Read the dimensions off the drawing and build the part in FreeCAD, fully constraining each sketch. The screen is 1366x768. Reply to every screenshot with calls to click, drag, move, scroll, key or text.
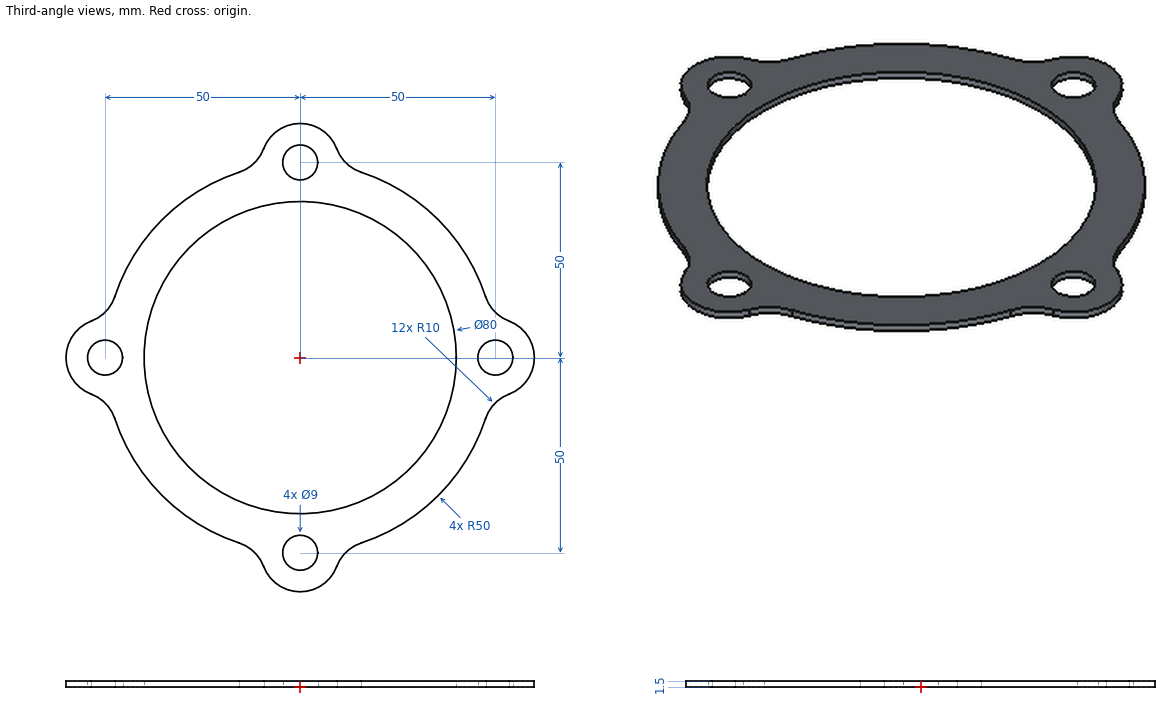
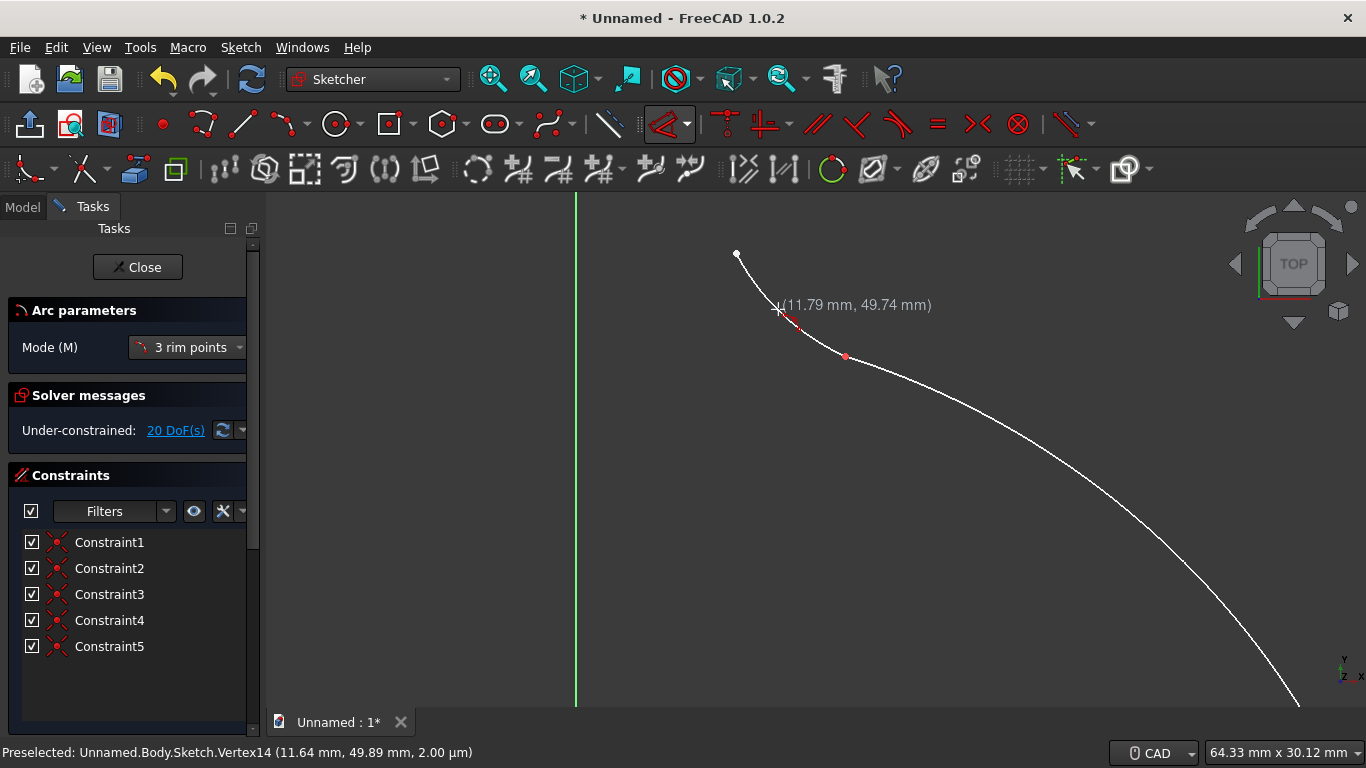
scroll(781, 309, down, 9)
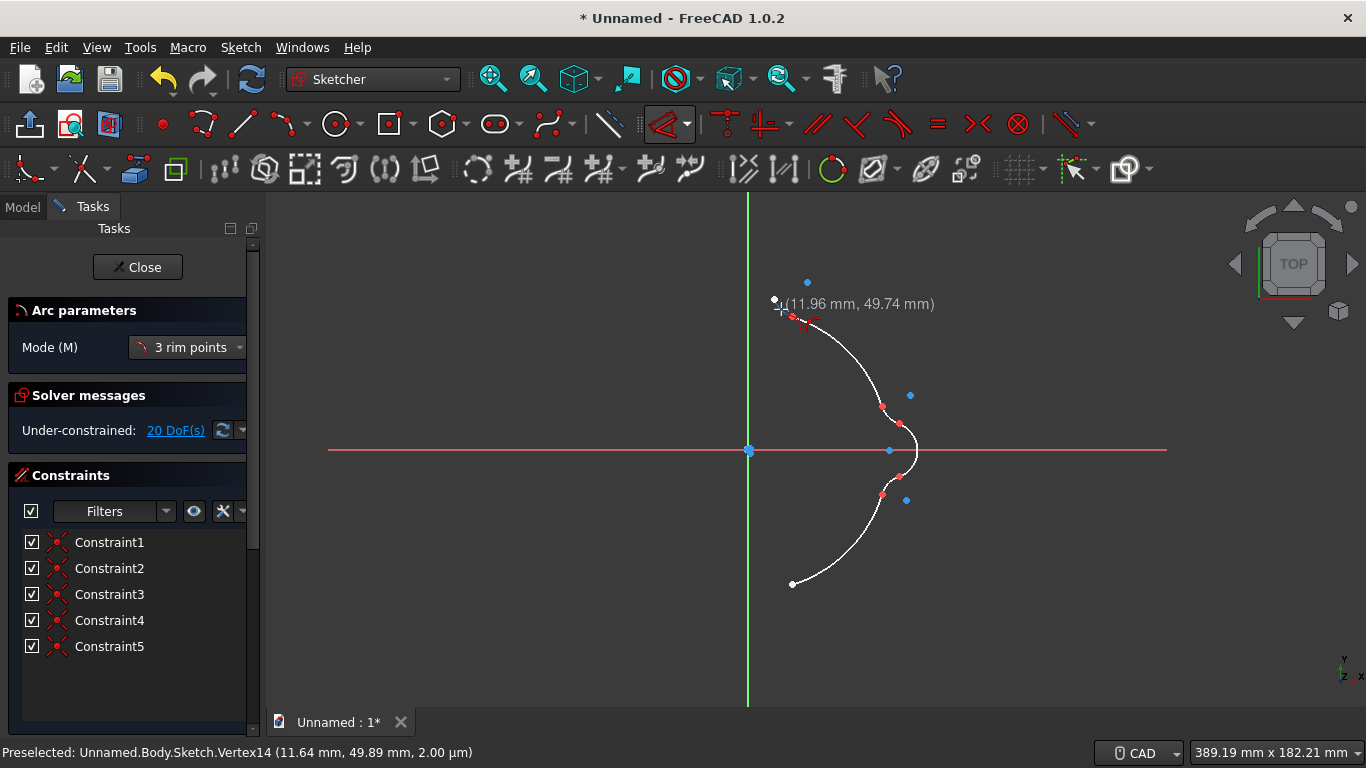
click(774, 300)
click(721, 299)
click(734, 284)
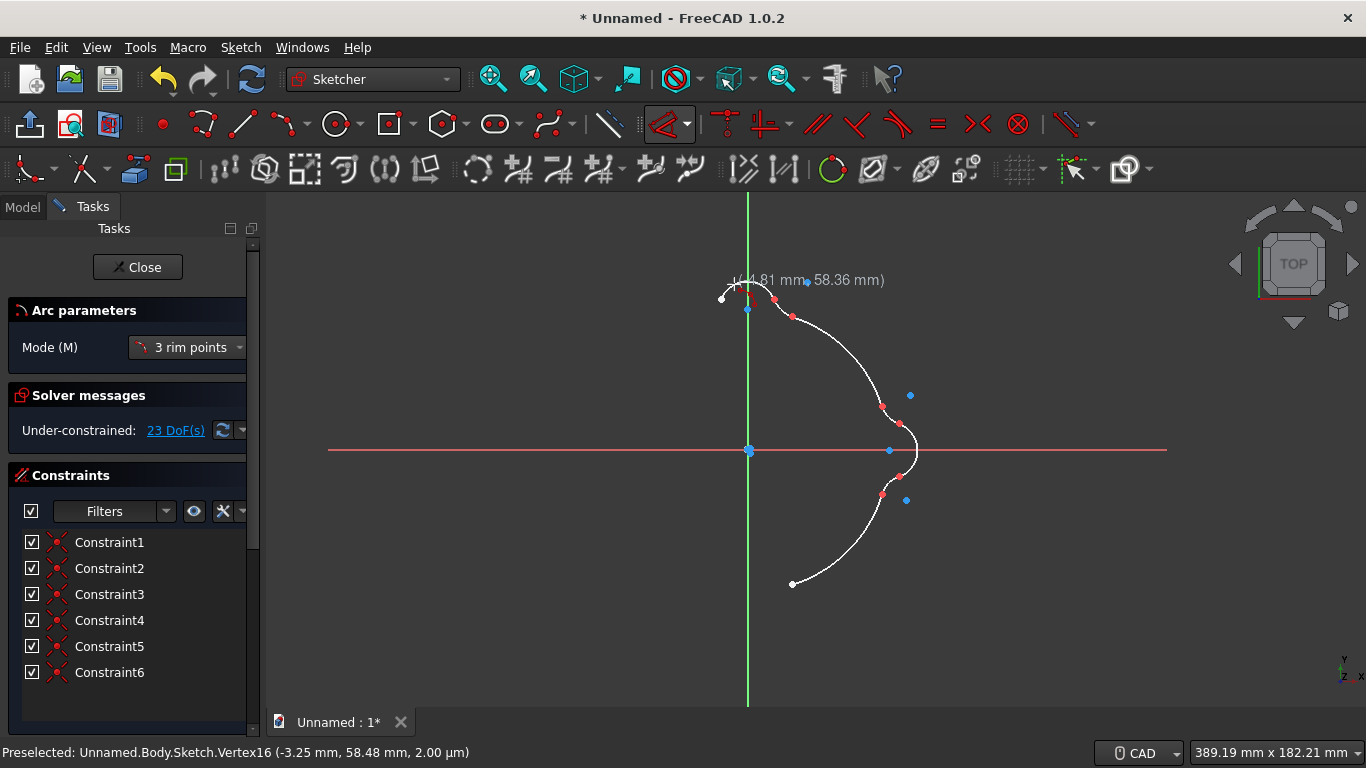
click(721, 300)
click(703, 316)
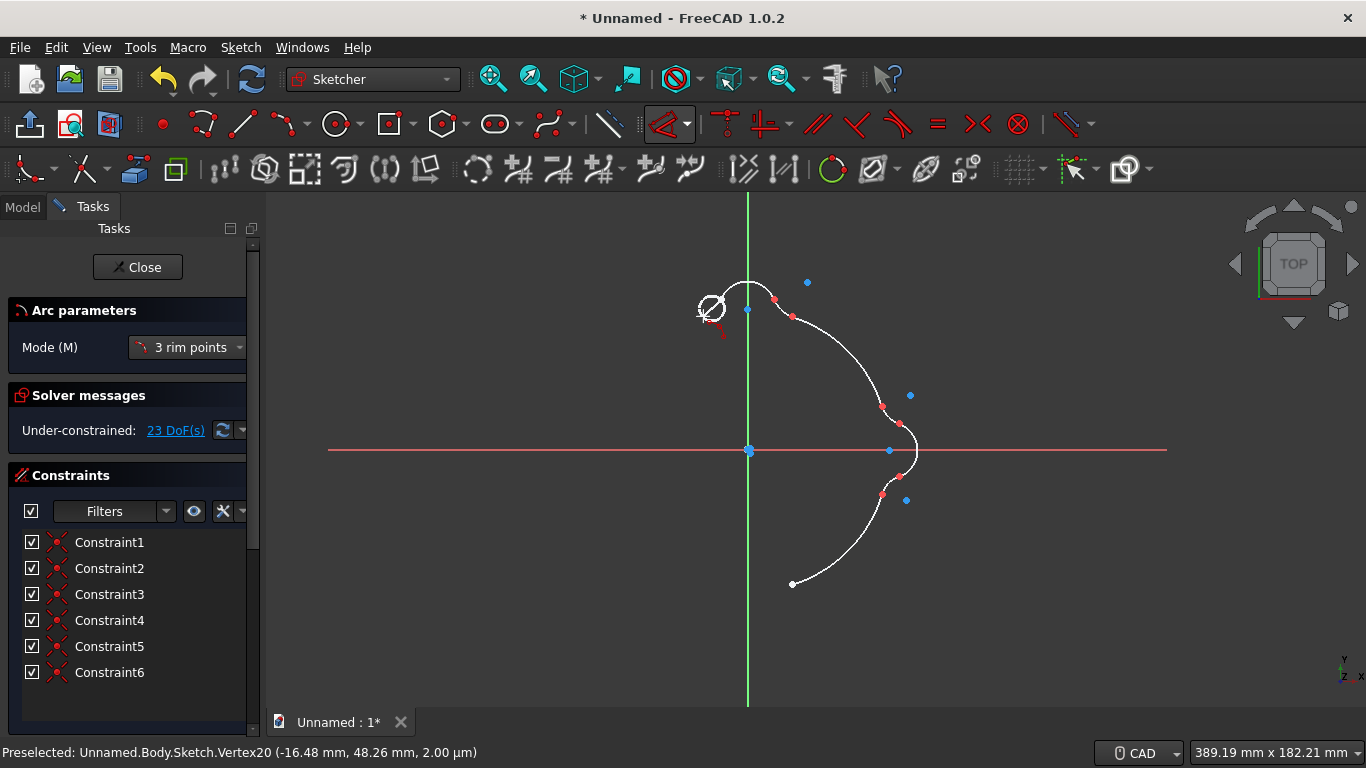
scroll(714, 309, up, 9)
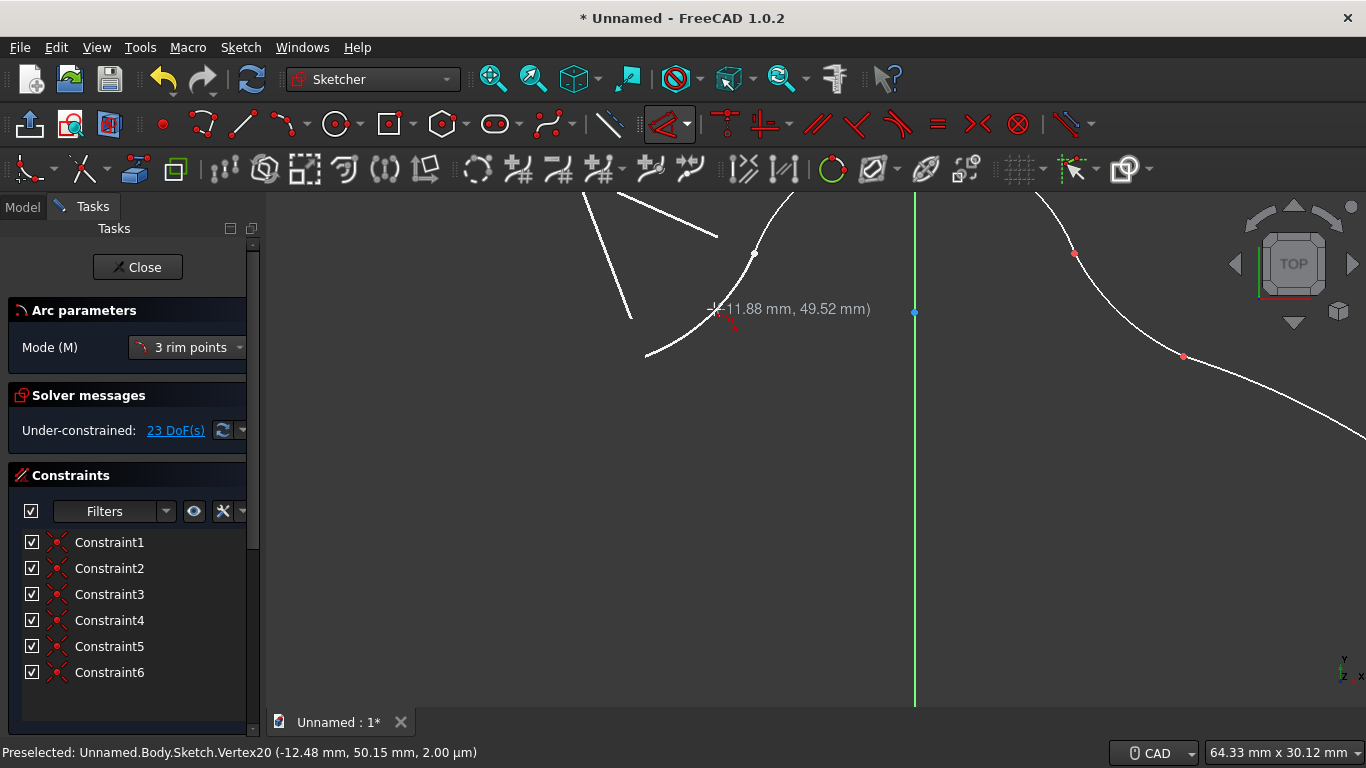
click(713, 309)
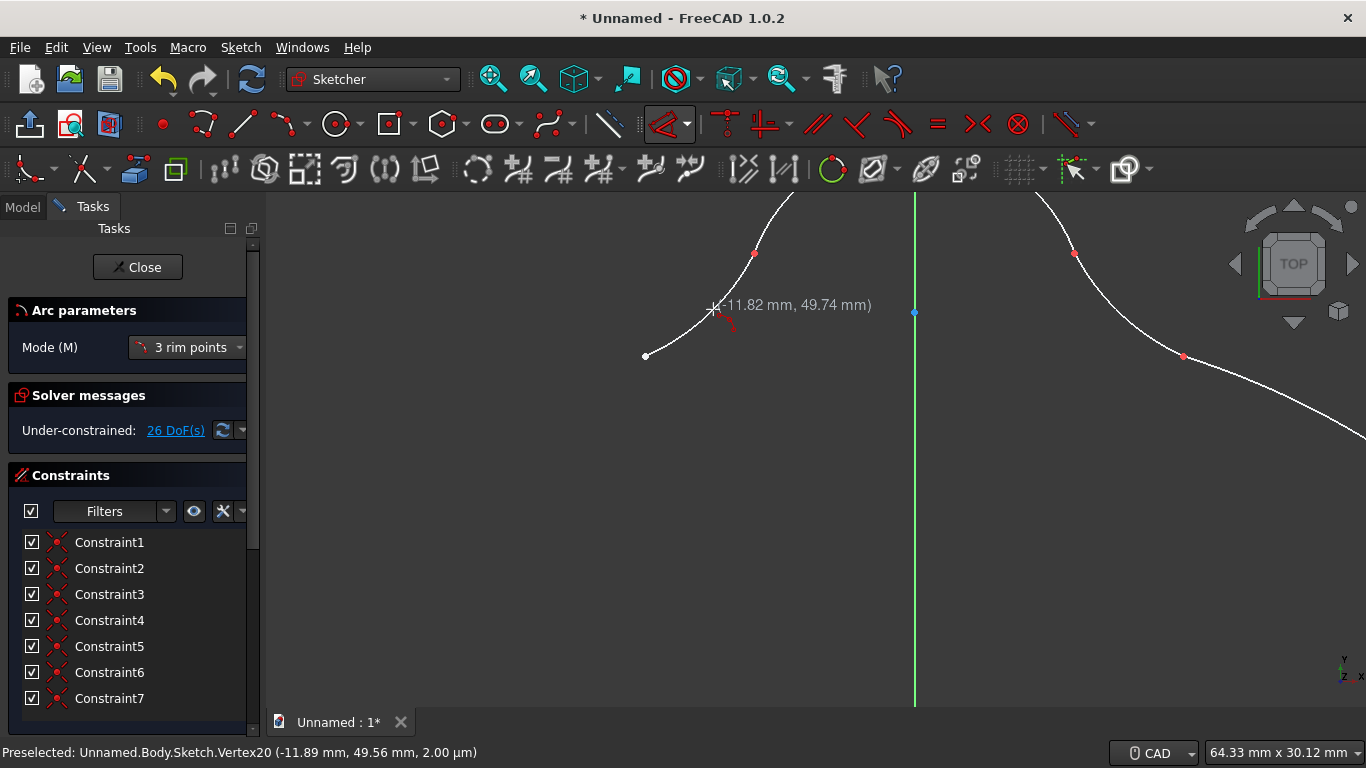
scroll(714, 309, down, 9)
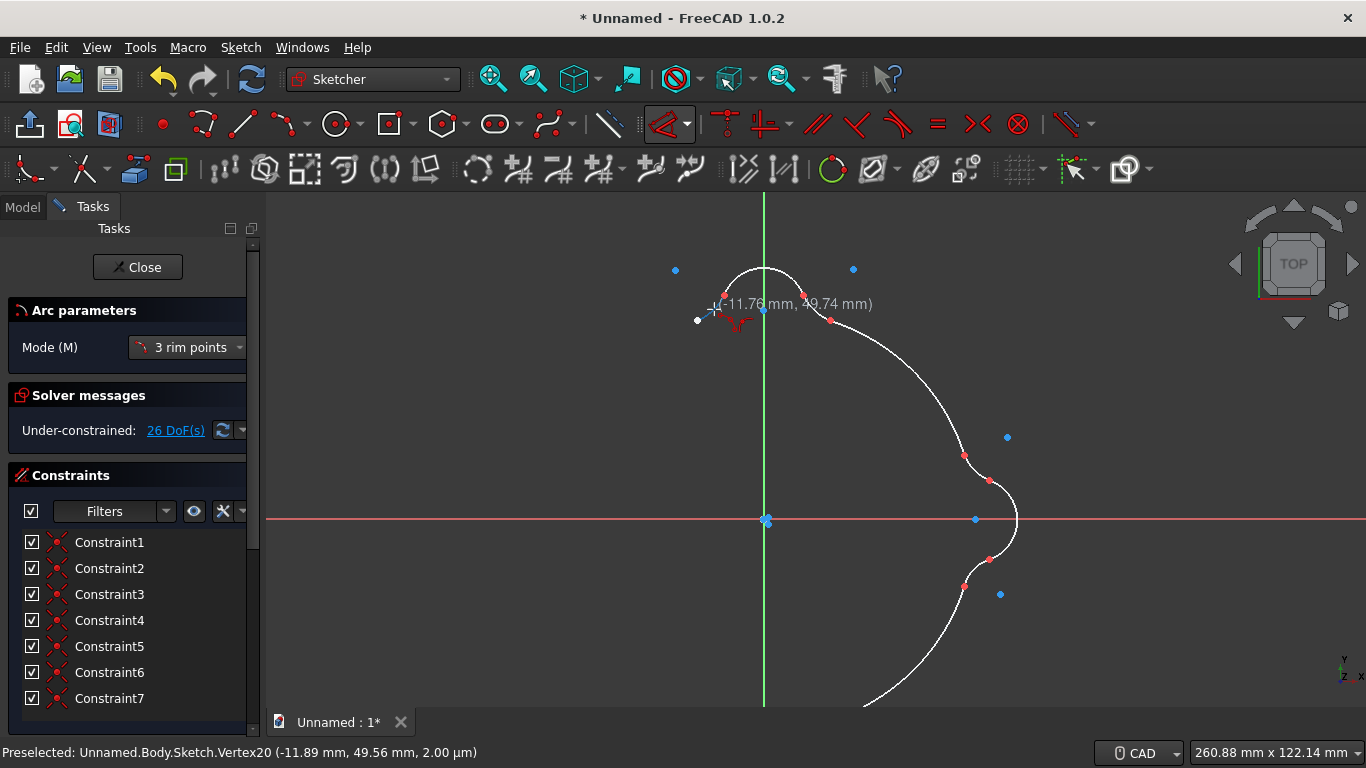
click(703, 317)
click(613, 406)
click(648, 350)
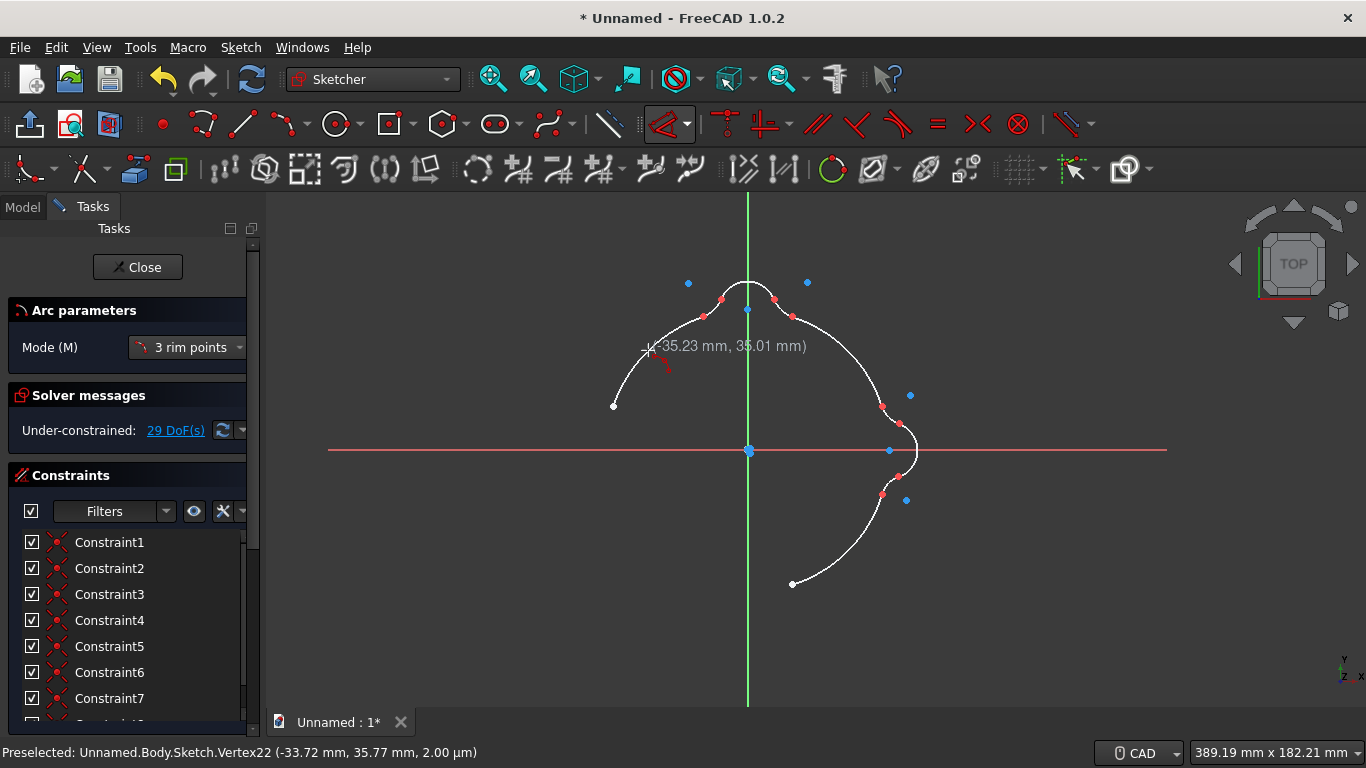
click(613, 407)
click(596, 423)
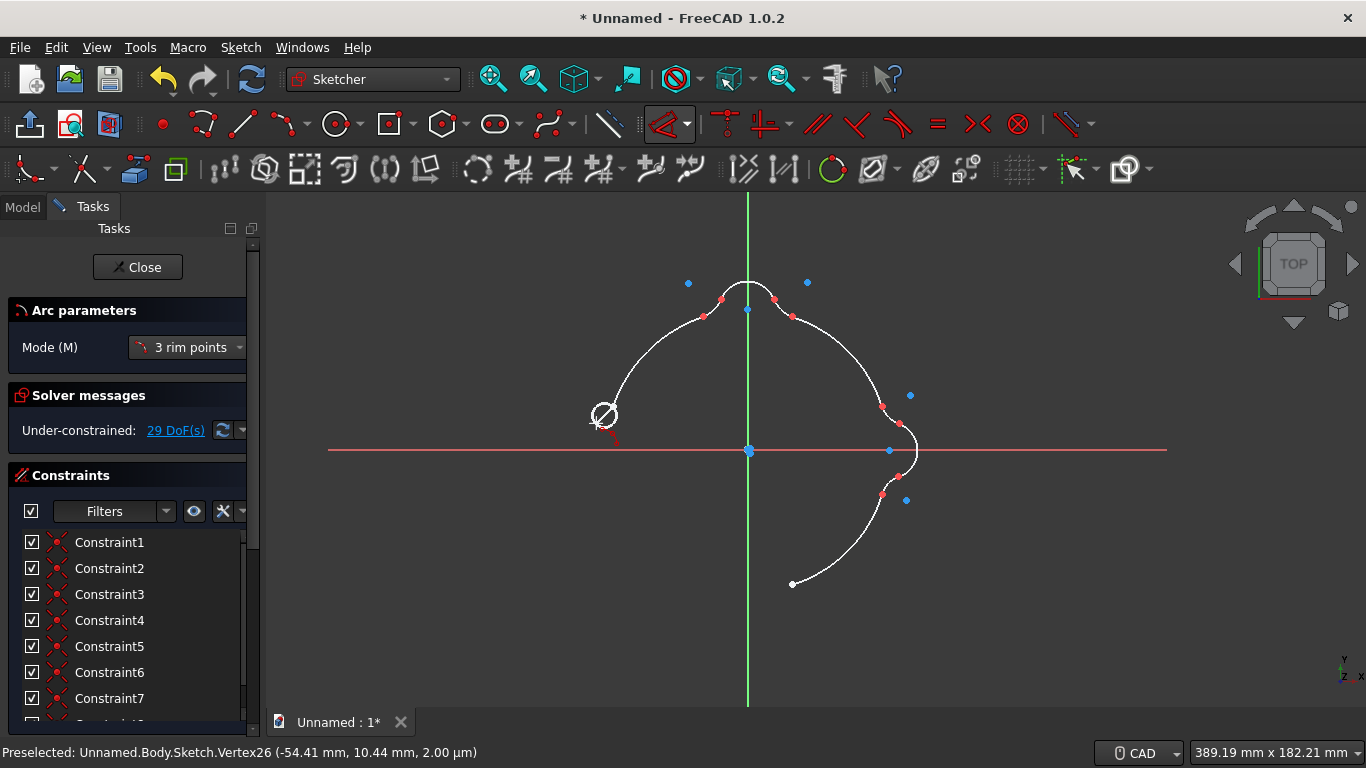
scroll(607, 417, up, 9)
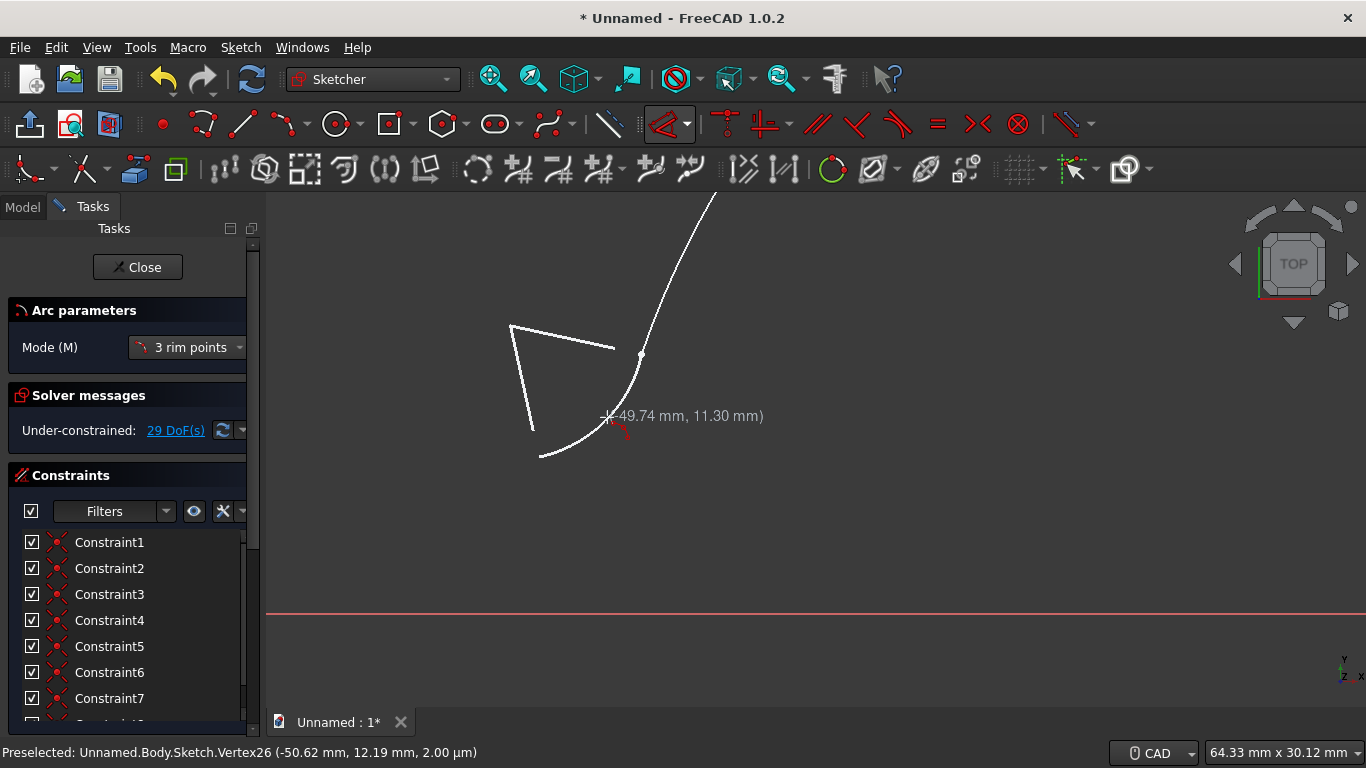
click(605, 412)